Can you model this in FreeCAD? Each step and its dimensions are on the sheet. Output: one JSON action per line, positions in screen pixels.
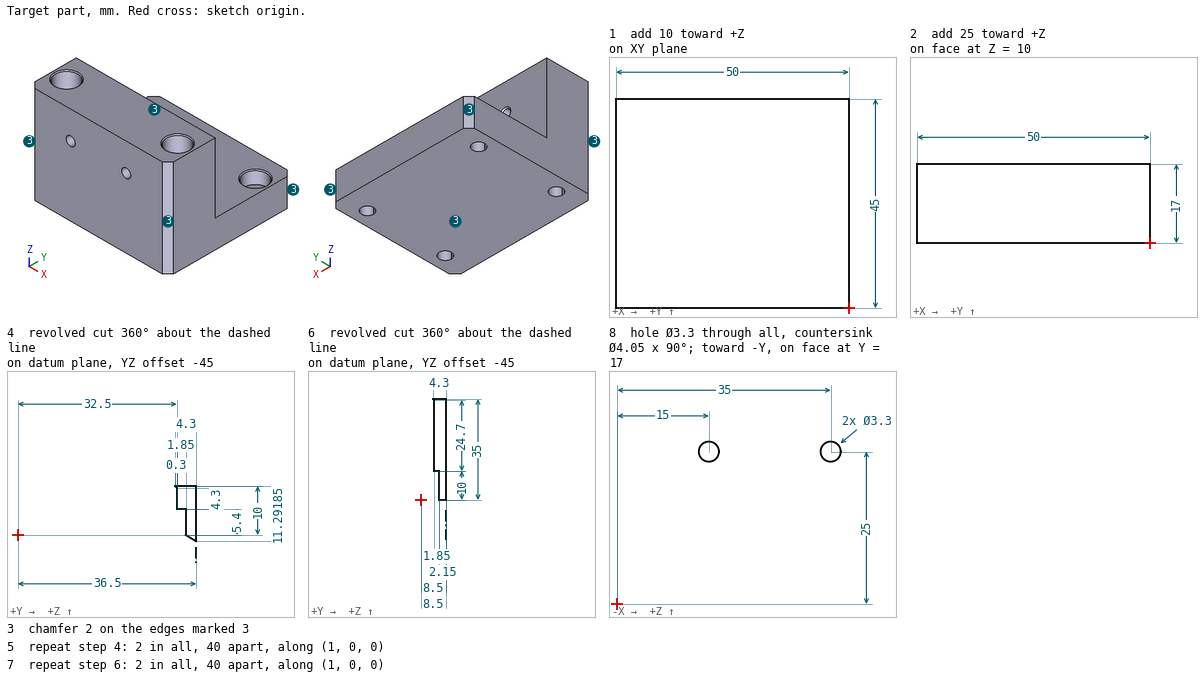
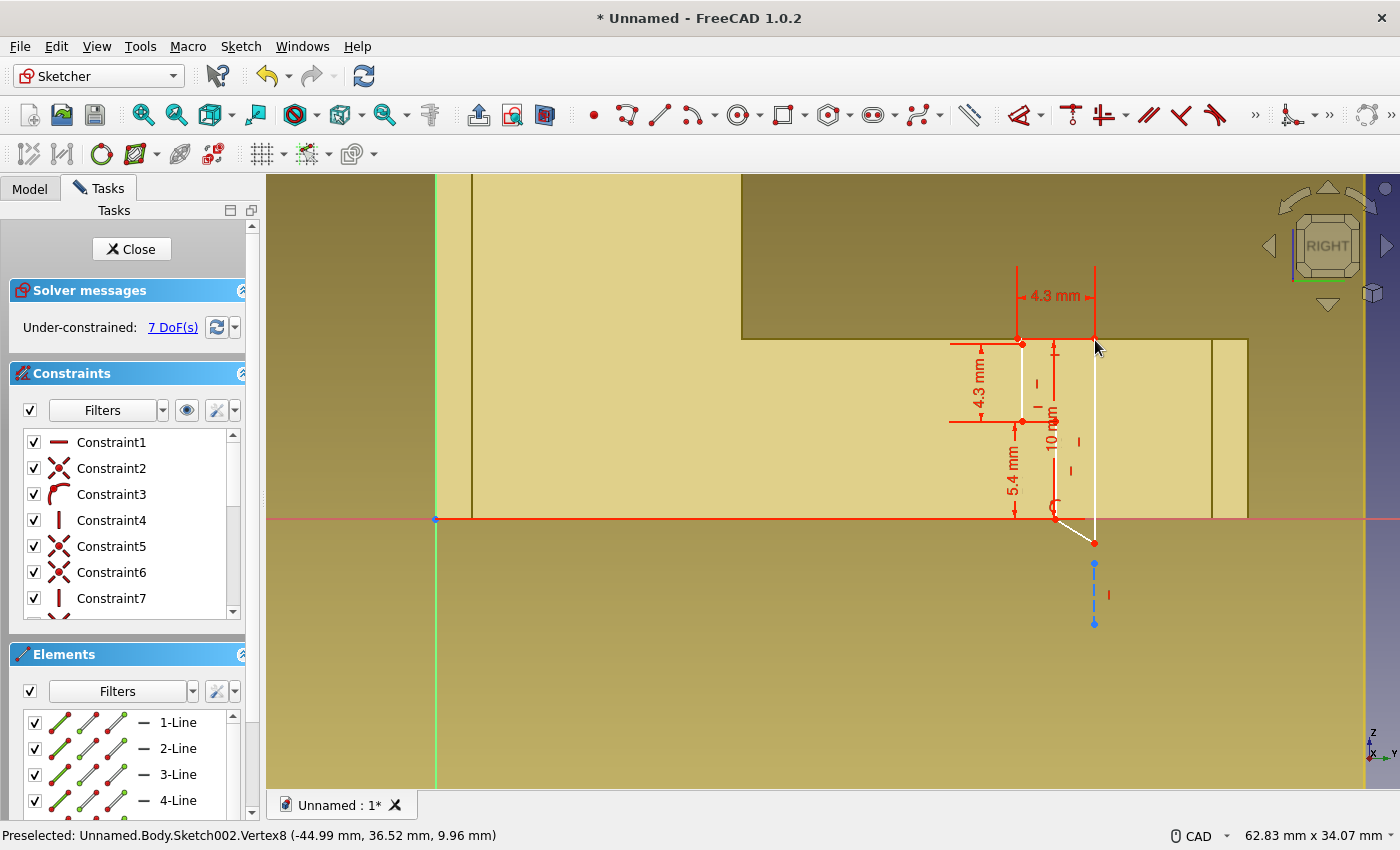
{"action": "scroll", "coordinate": [1032, 422], "scroll_direction": "up", "scroll_amount": 2}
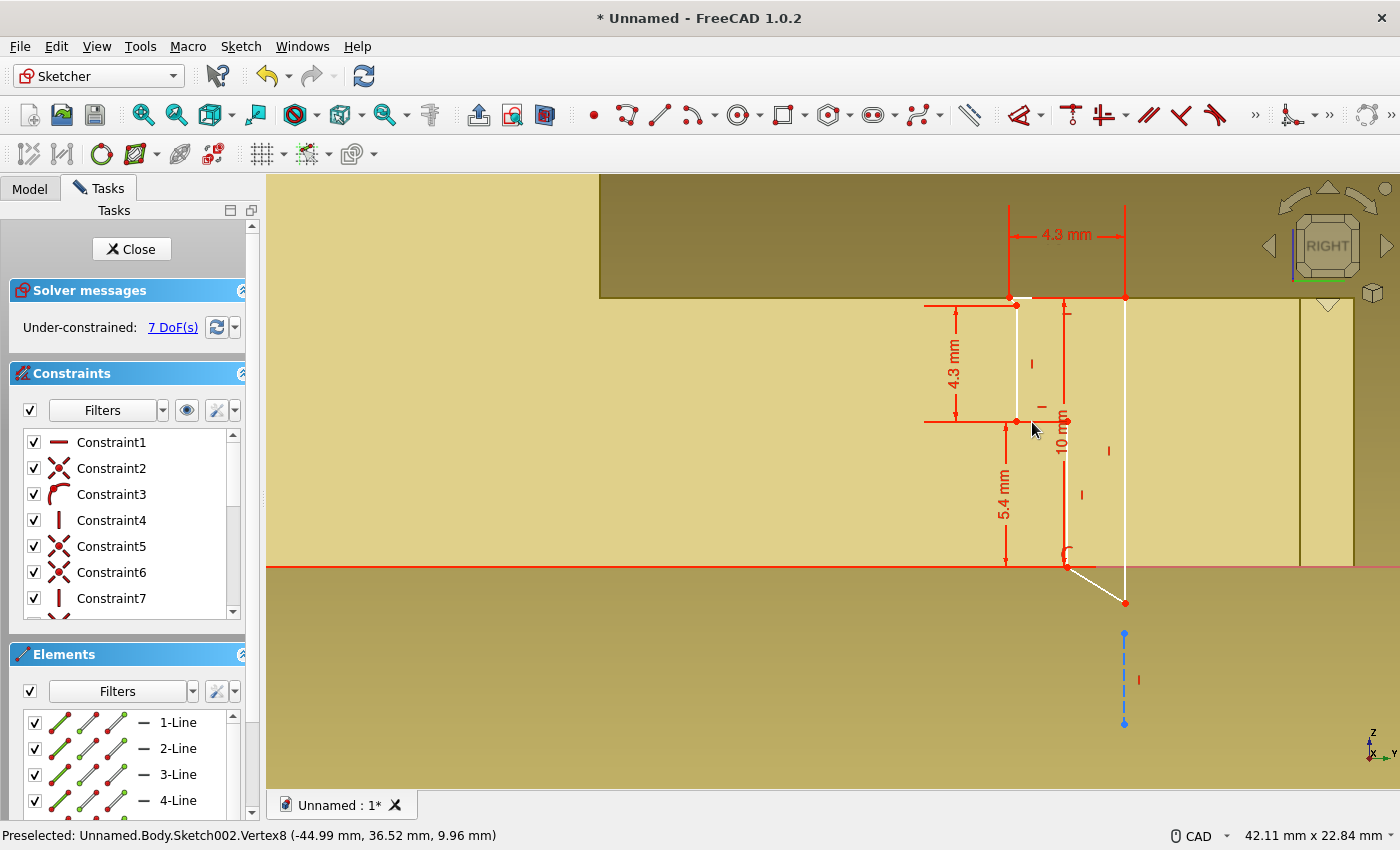
{"action": "left_click", "coordinate": [1032, 422]}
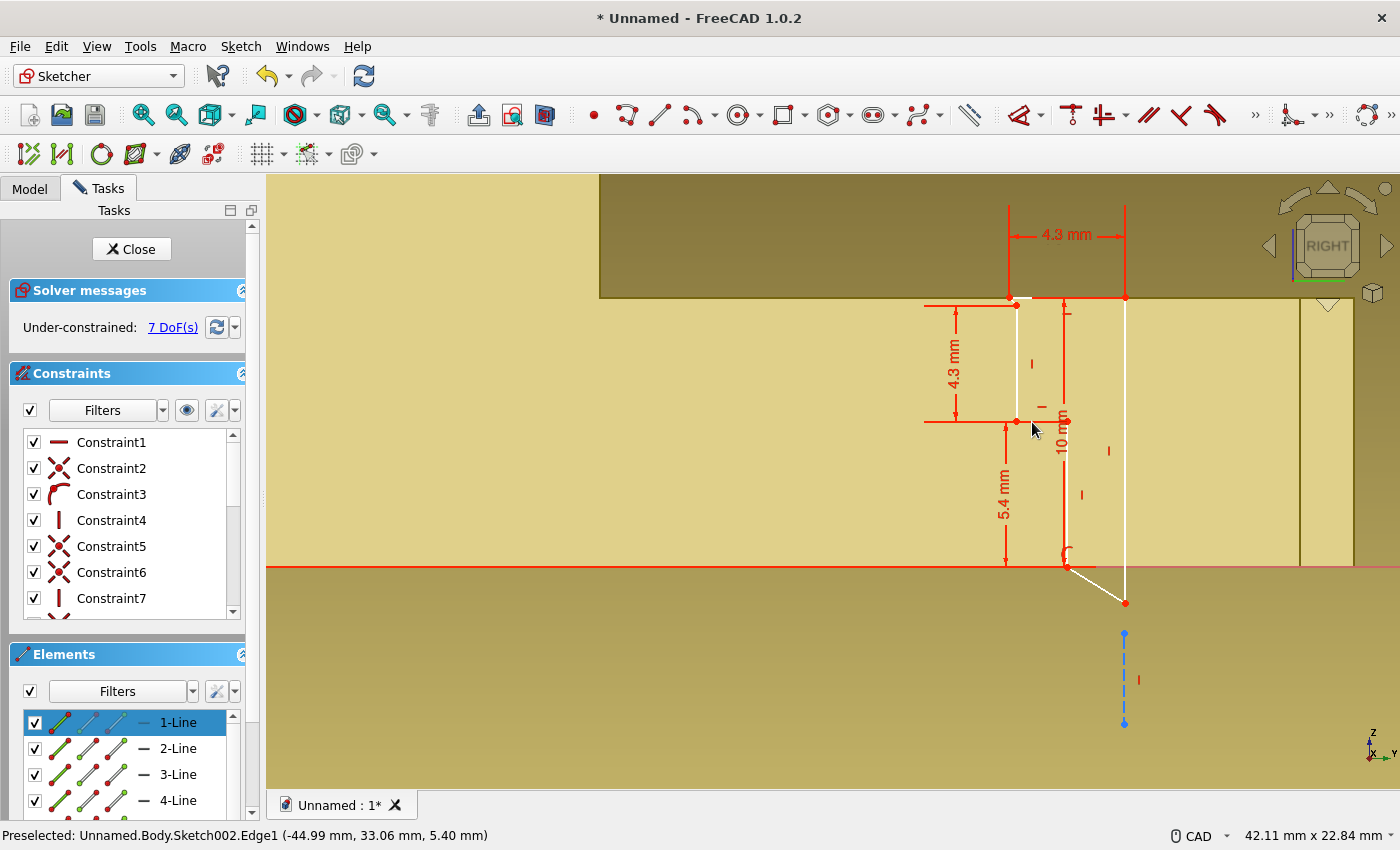
{"action": "key", "text": "l"}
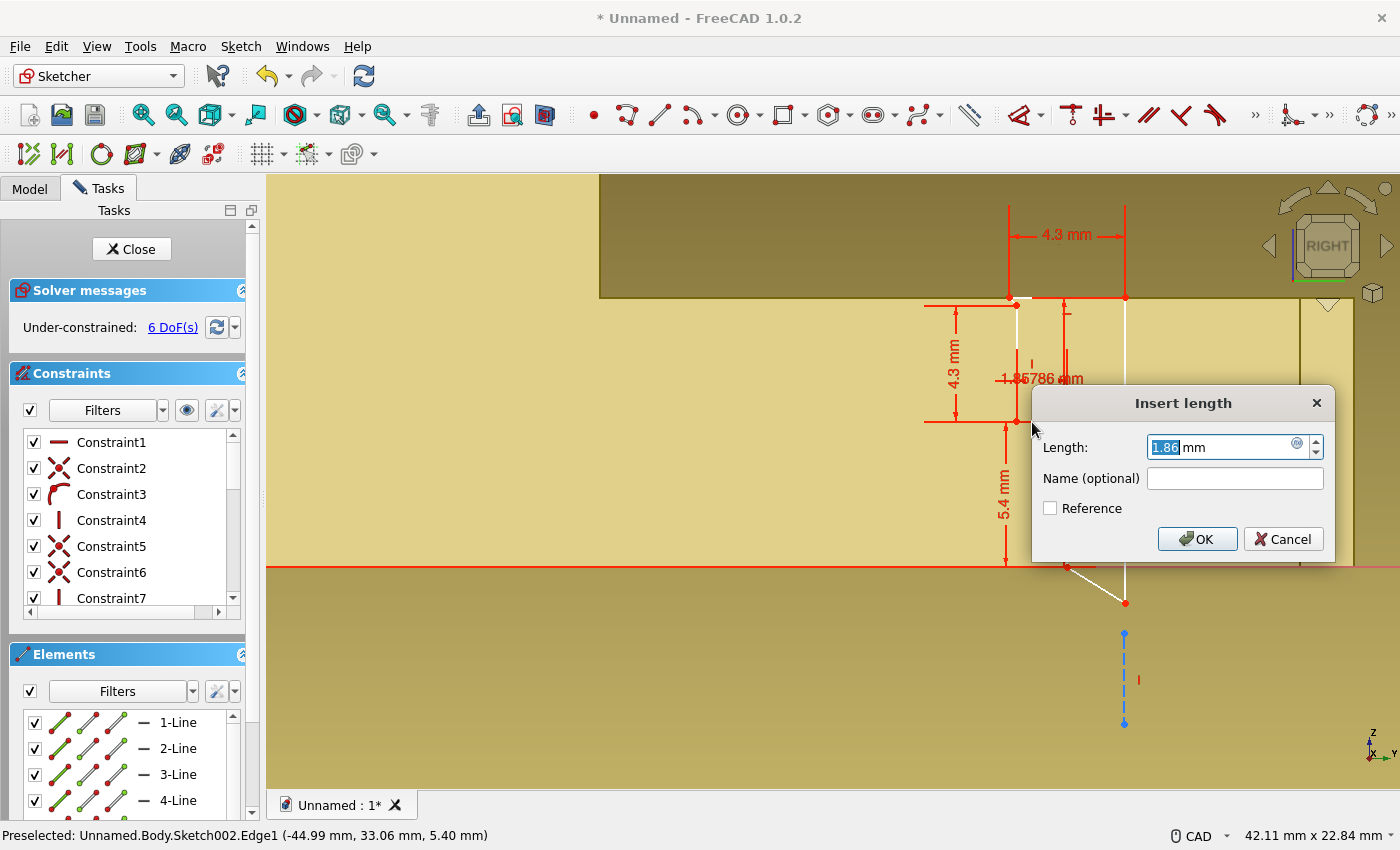
{"action": "type", "text": "1.85"}
{"action": "key", "text": "Return"}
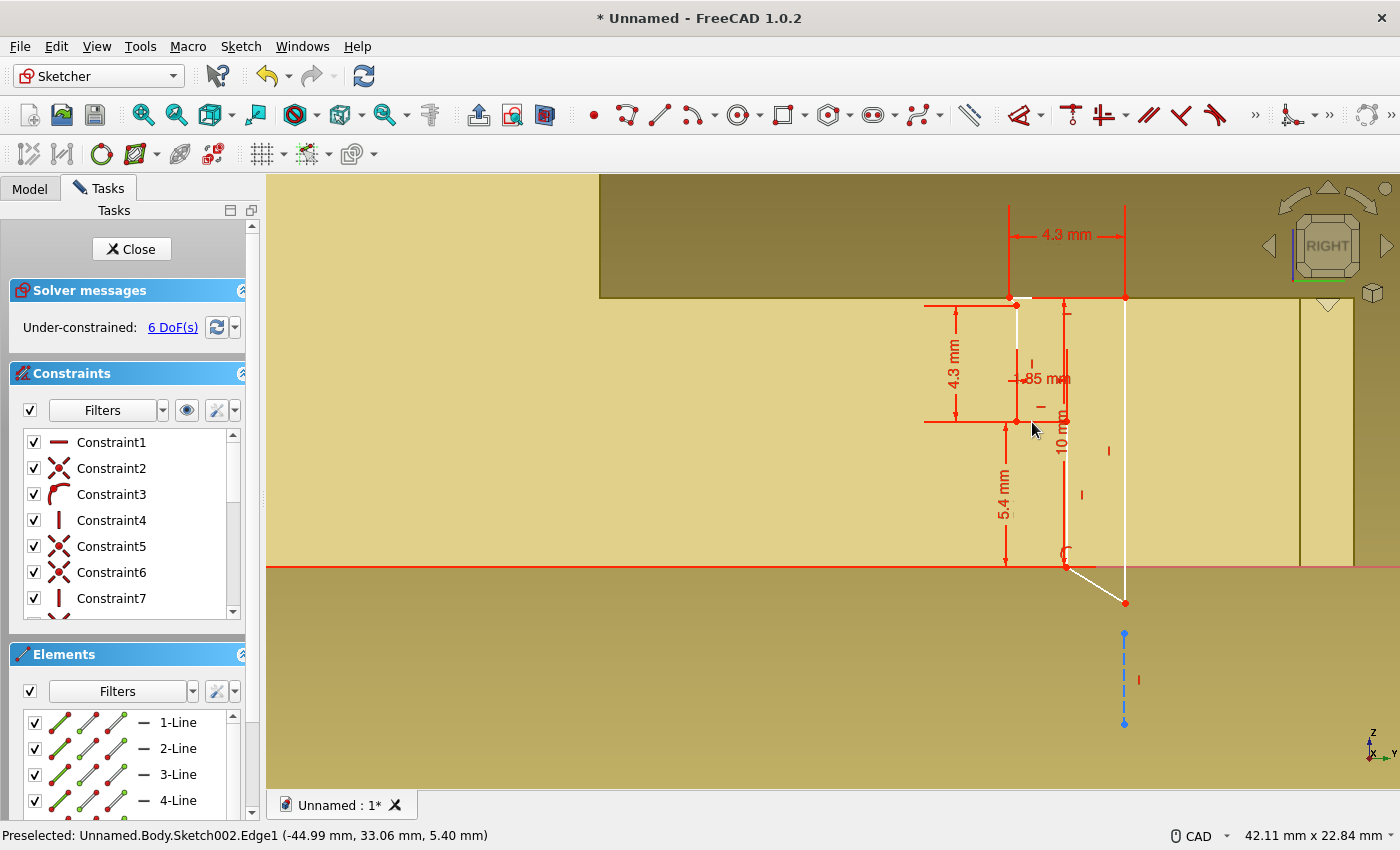
{"action": "scroll", "coordinate": [1014, 303], "scroll_direction": "up", "scroll_amount": 8}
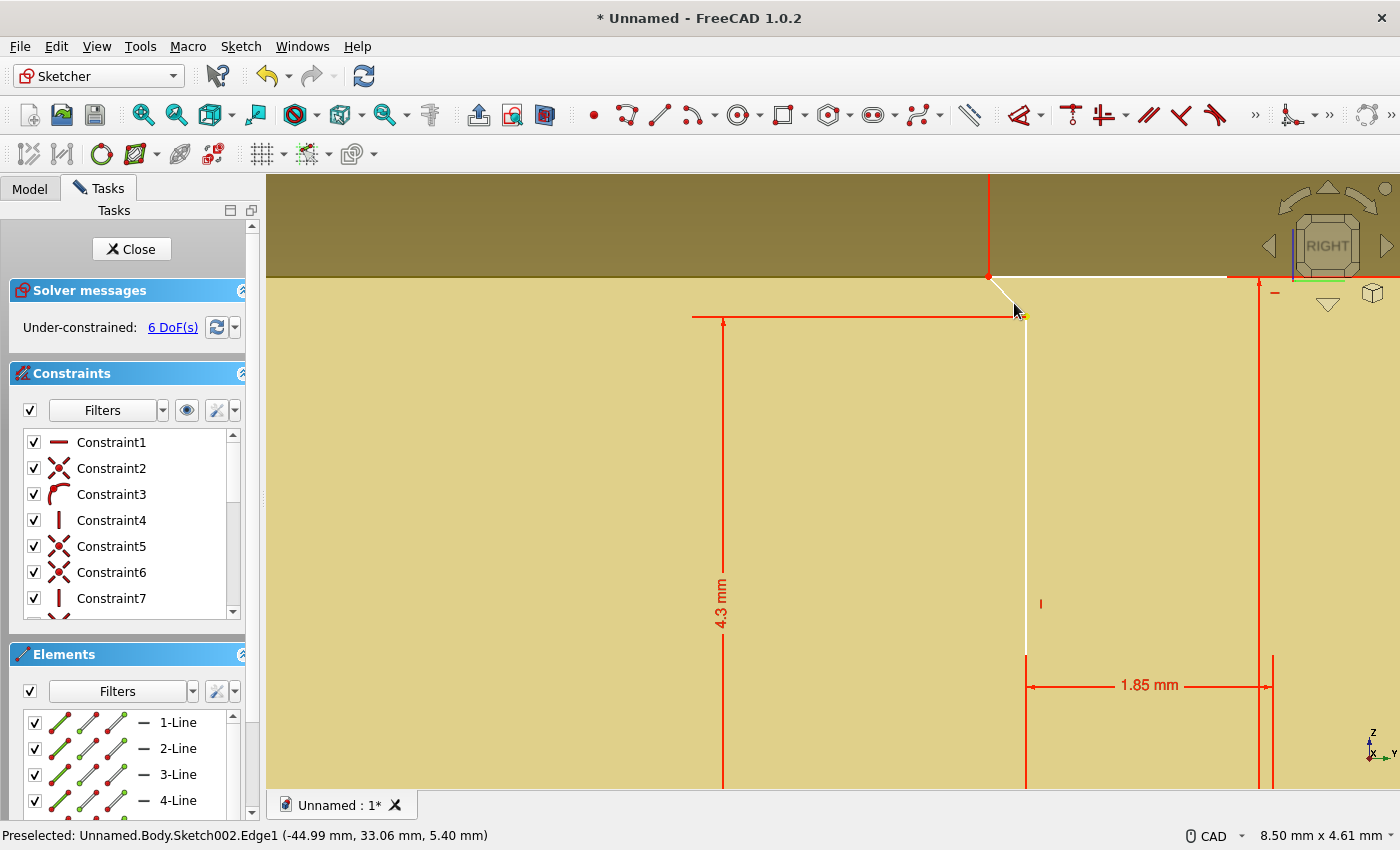
{"action": "left_click", "coordinate": [1011, 301]}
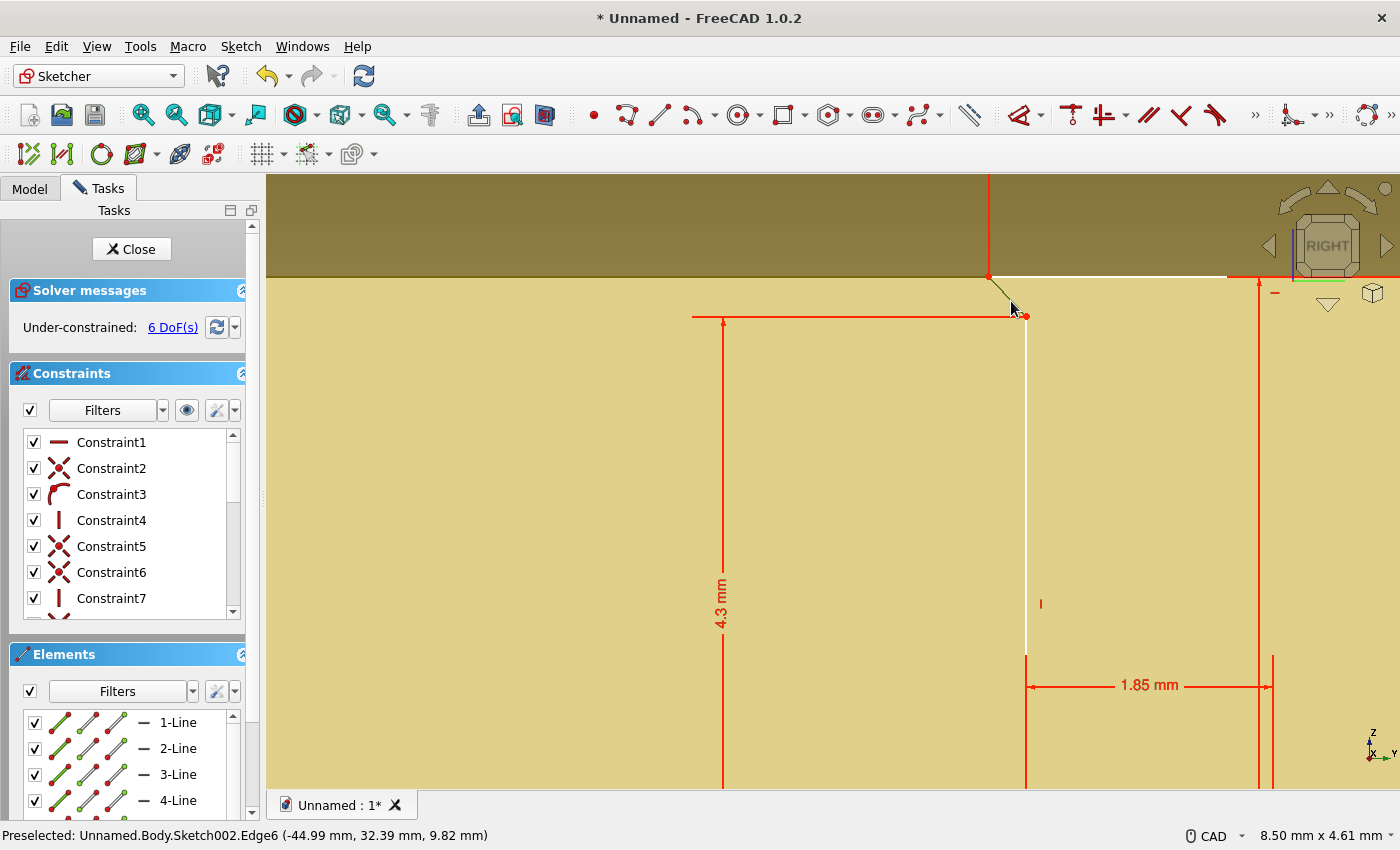
{"action": "key", "text": "l"}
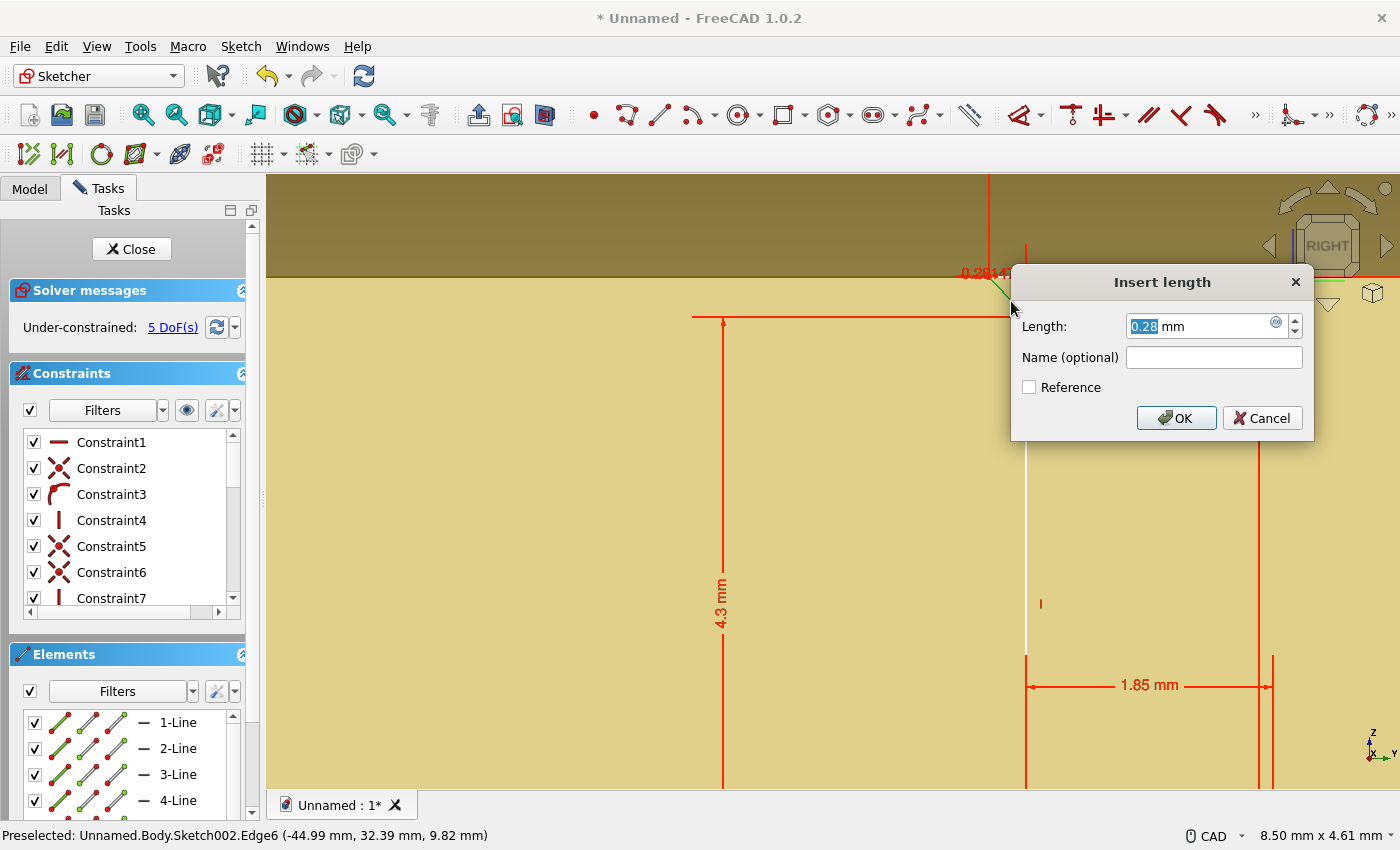
{"action": "type", "text": "0.3"}
{"action": "key", "text": "Return"}